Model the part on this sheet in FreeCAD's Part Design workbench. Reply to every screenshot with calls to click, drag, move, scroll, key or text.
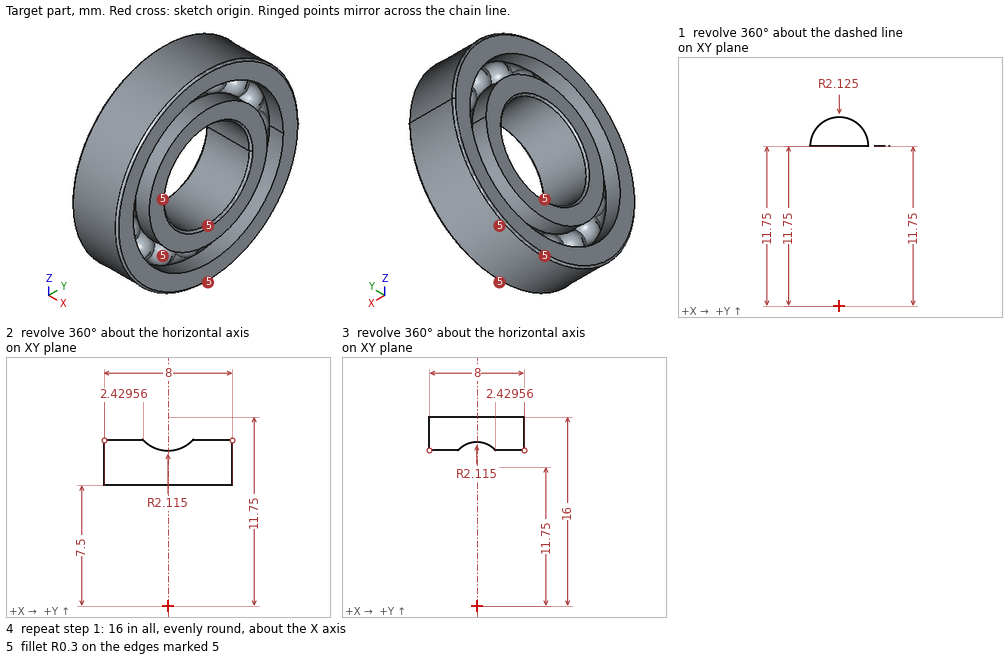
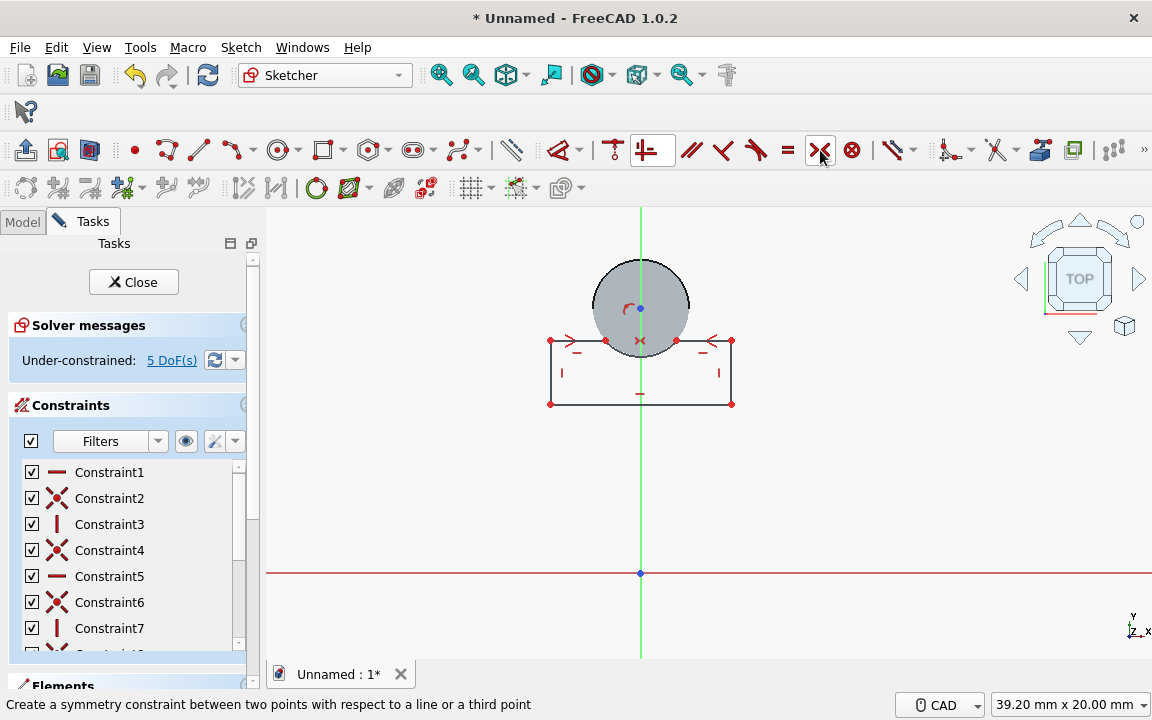
click(558, 150)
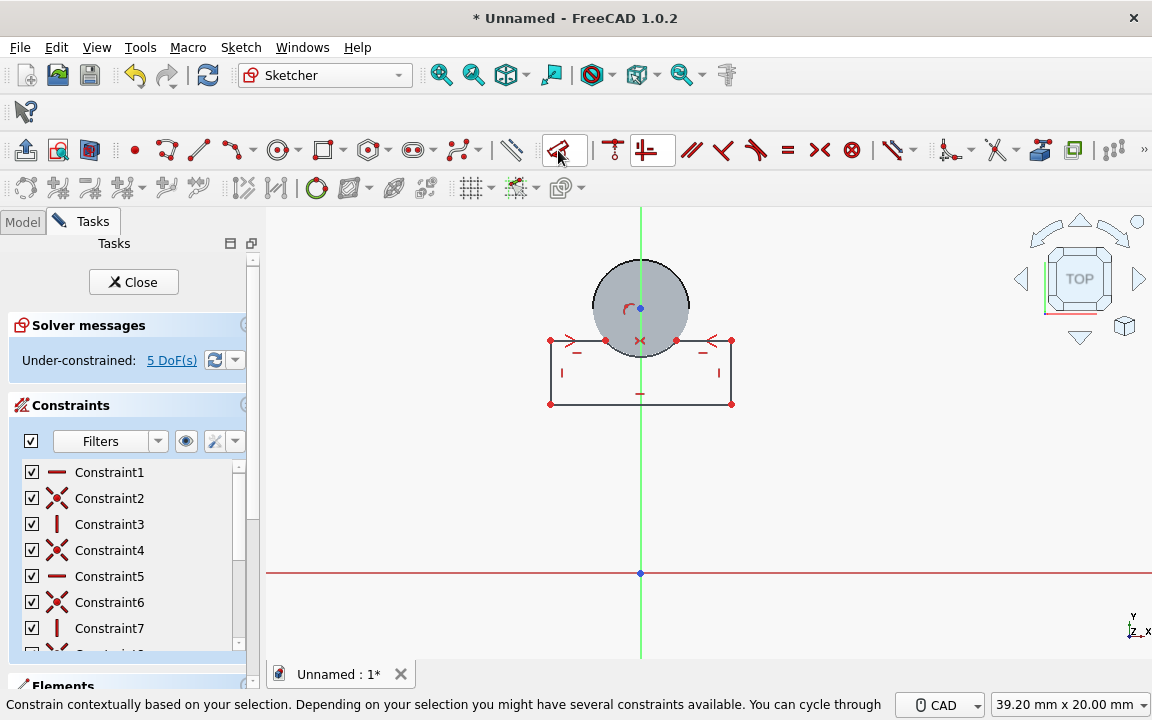
click(625, 354)
click(614, 384)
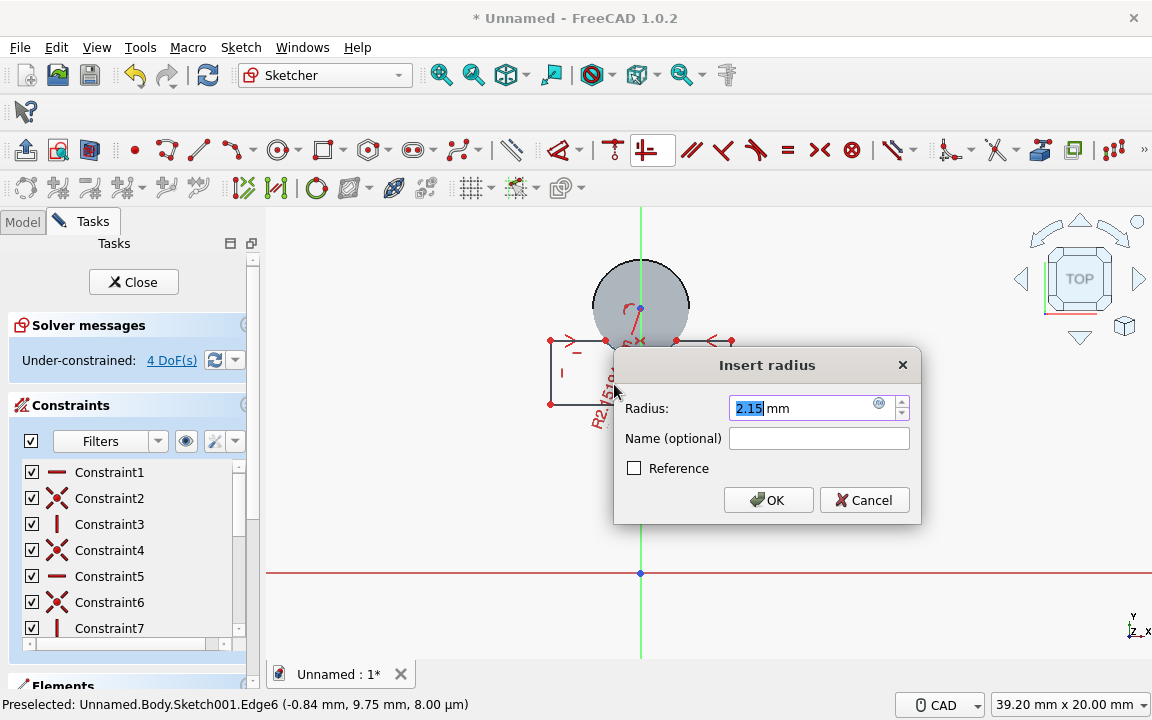
text(2.115)
key(Return)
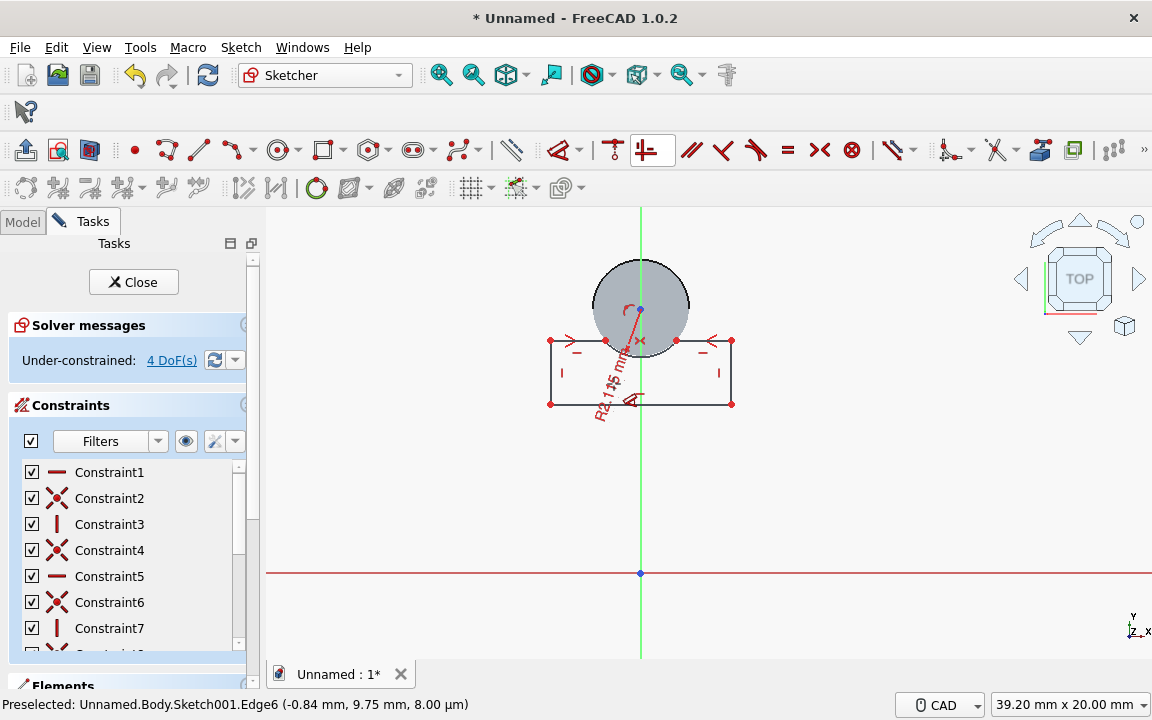
click(605, 405)
click(704, 371)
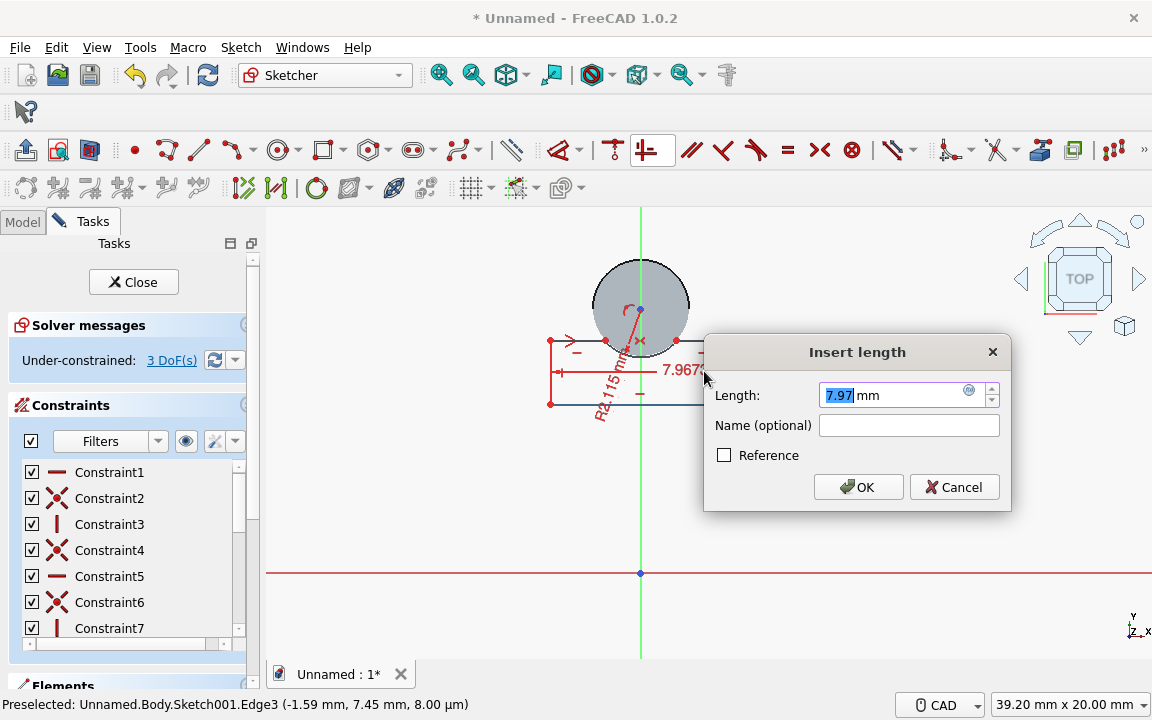
text(8)
key(Return)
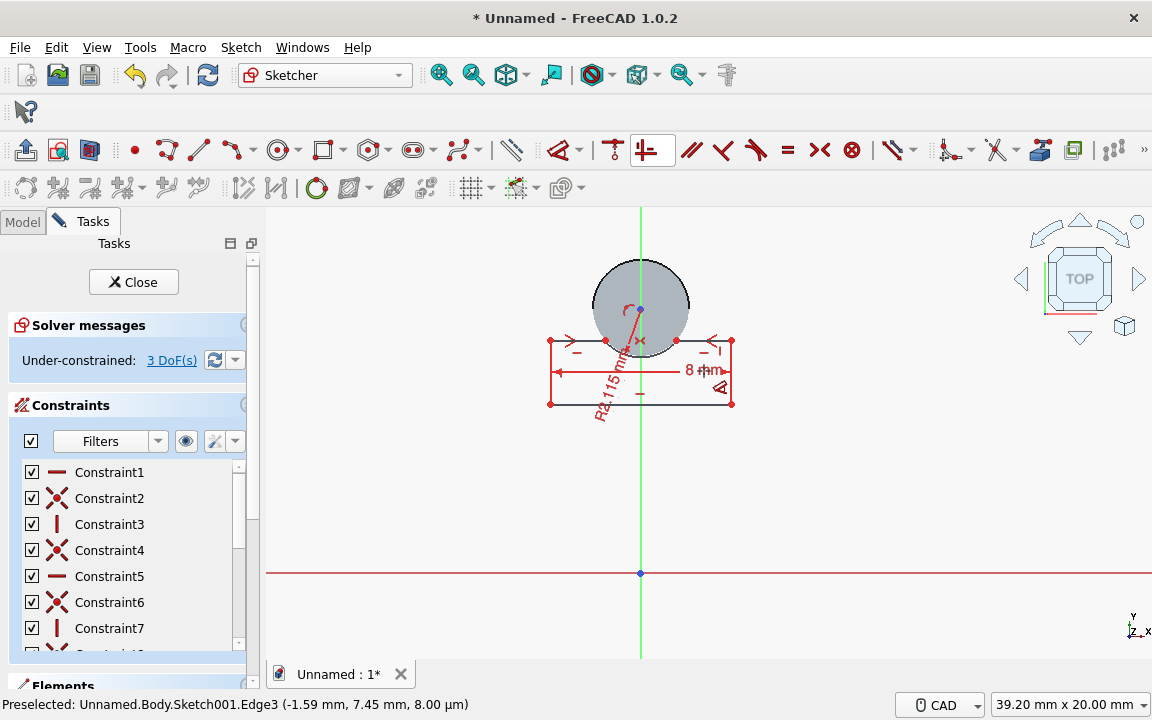
click(551, 405)
click(517, 489)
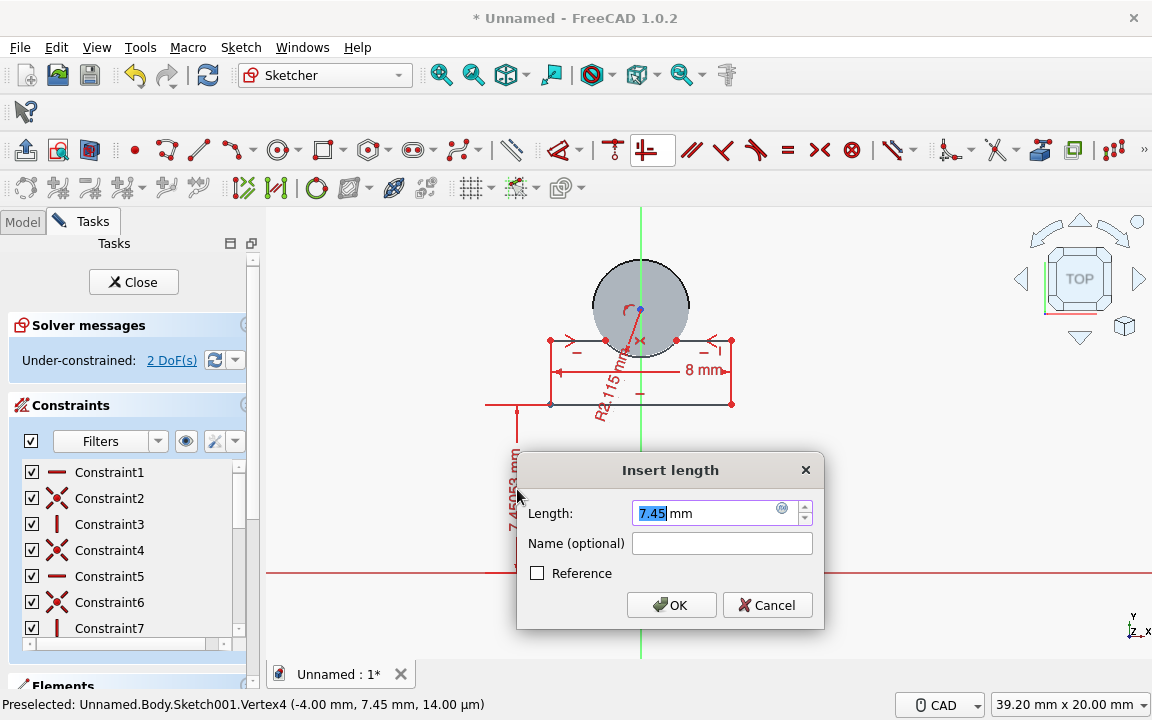
text(7.5)
key(Return)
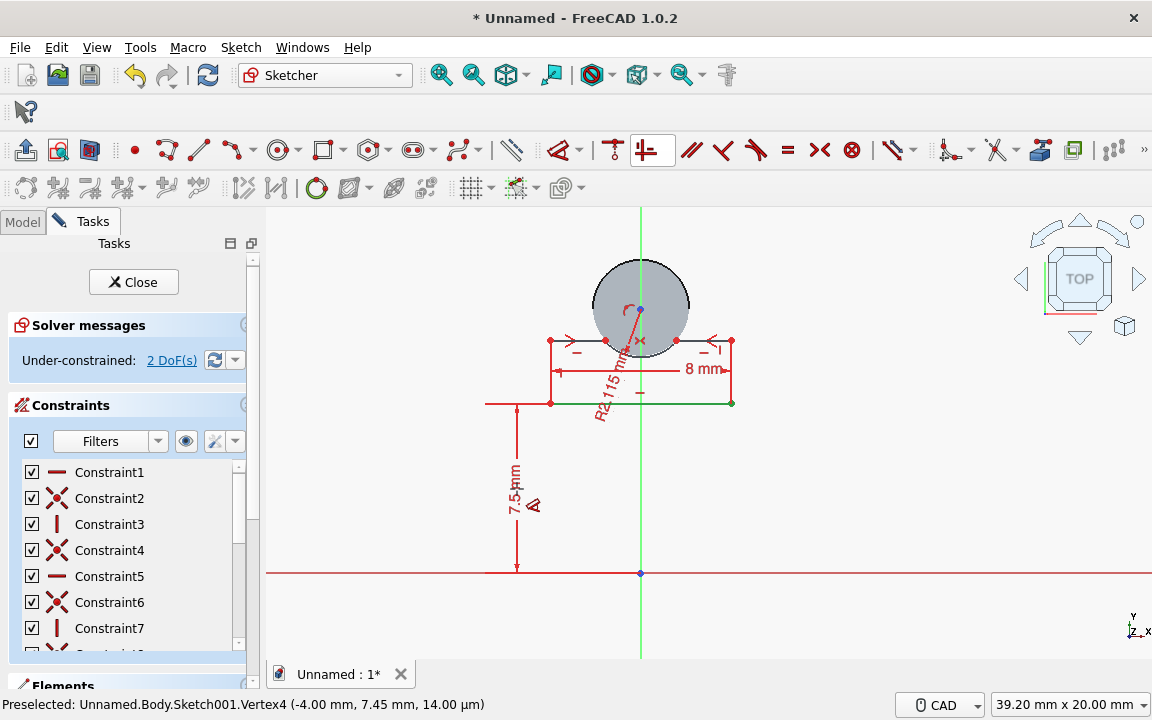
click(641, 310)
click(675, 441)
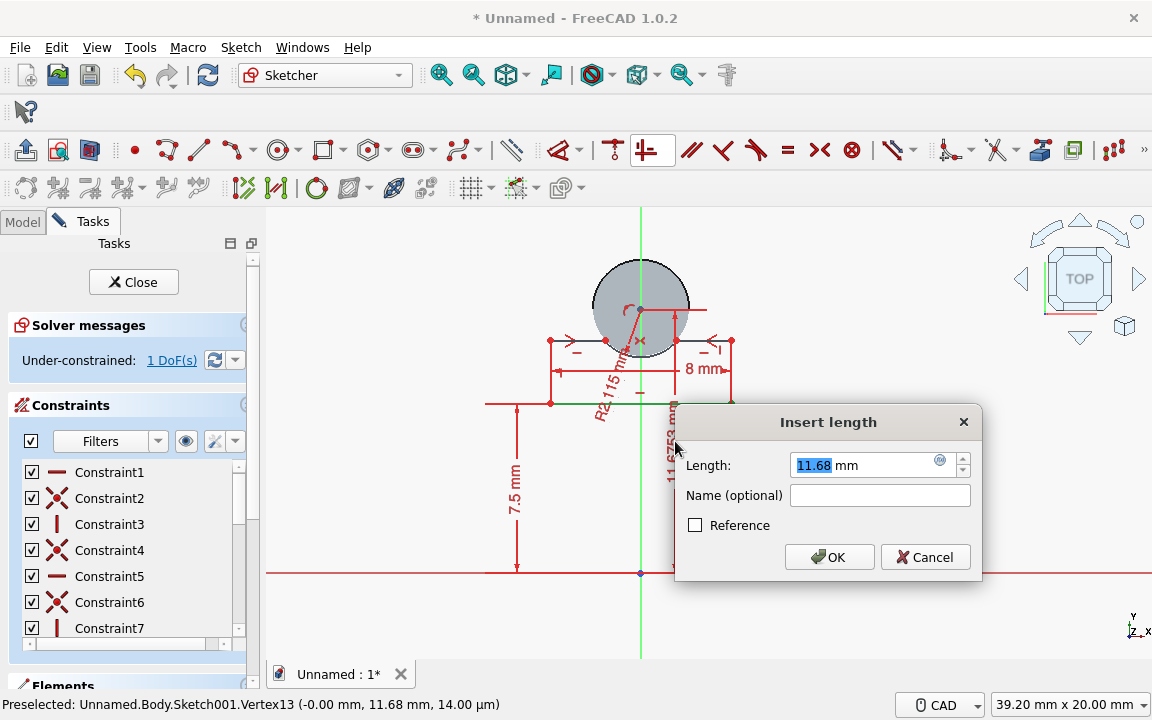
text(11.75)
key(Return)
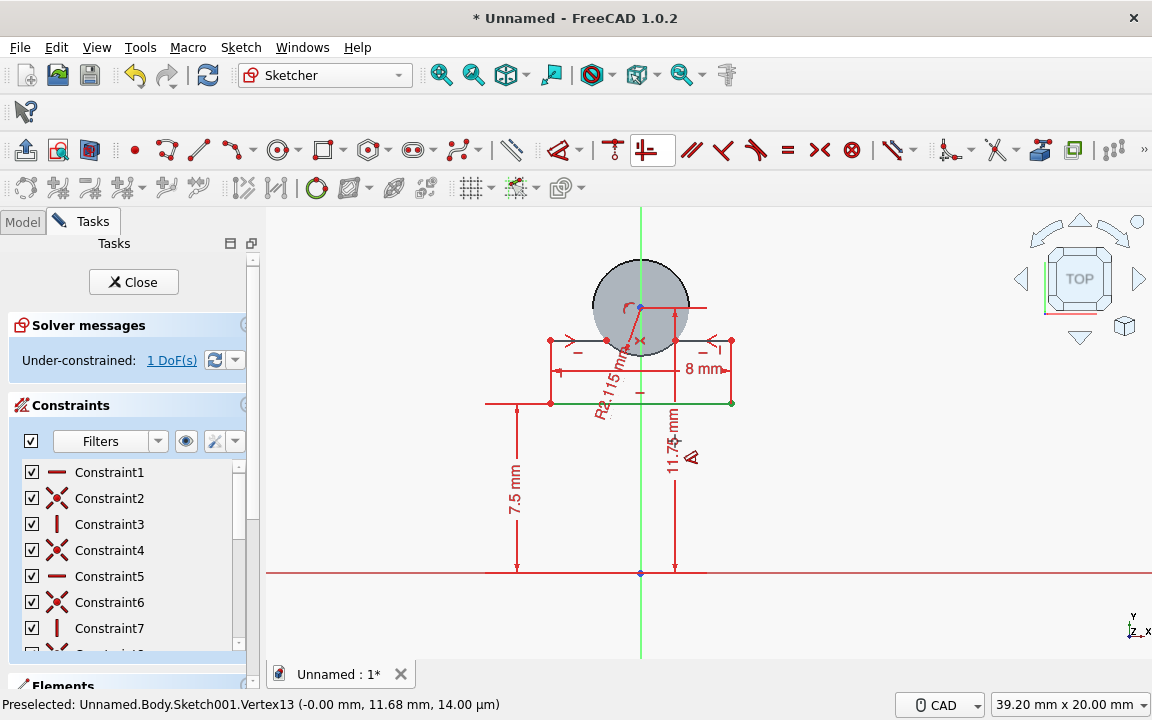
click(590, 341)
click(579, 307)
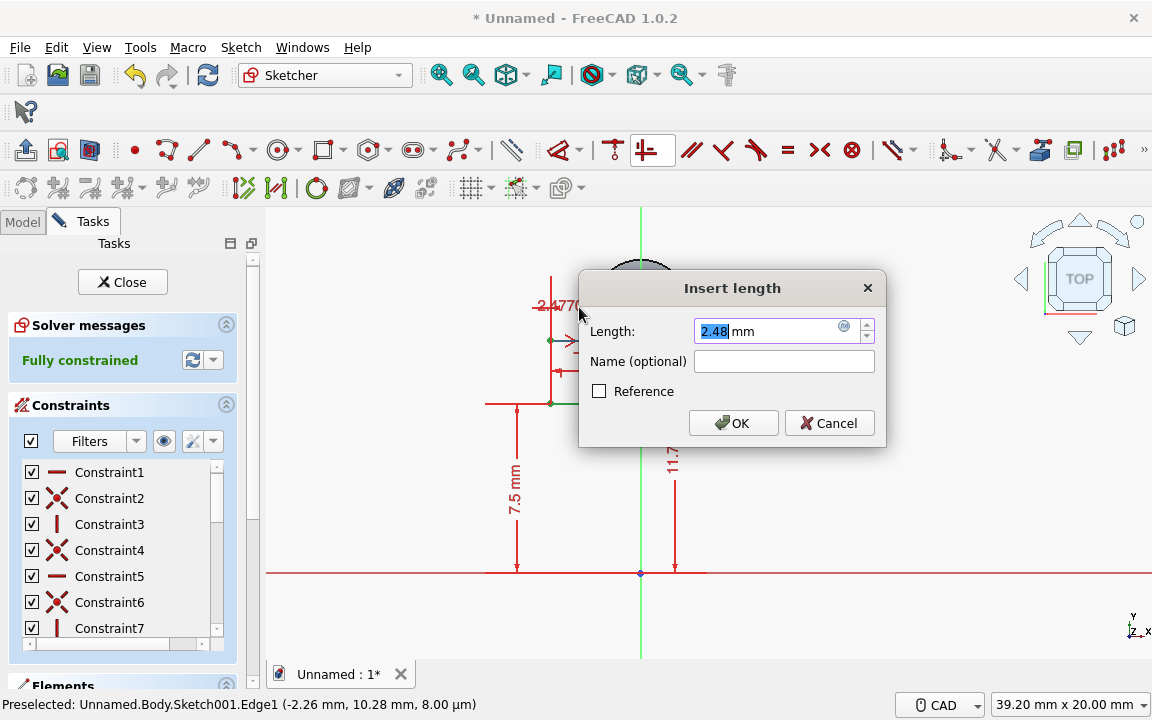
text(2.42956)
key(Return)
key(Escape)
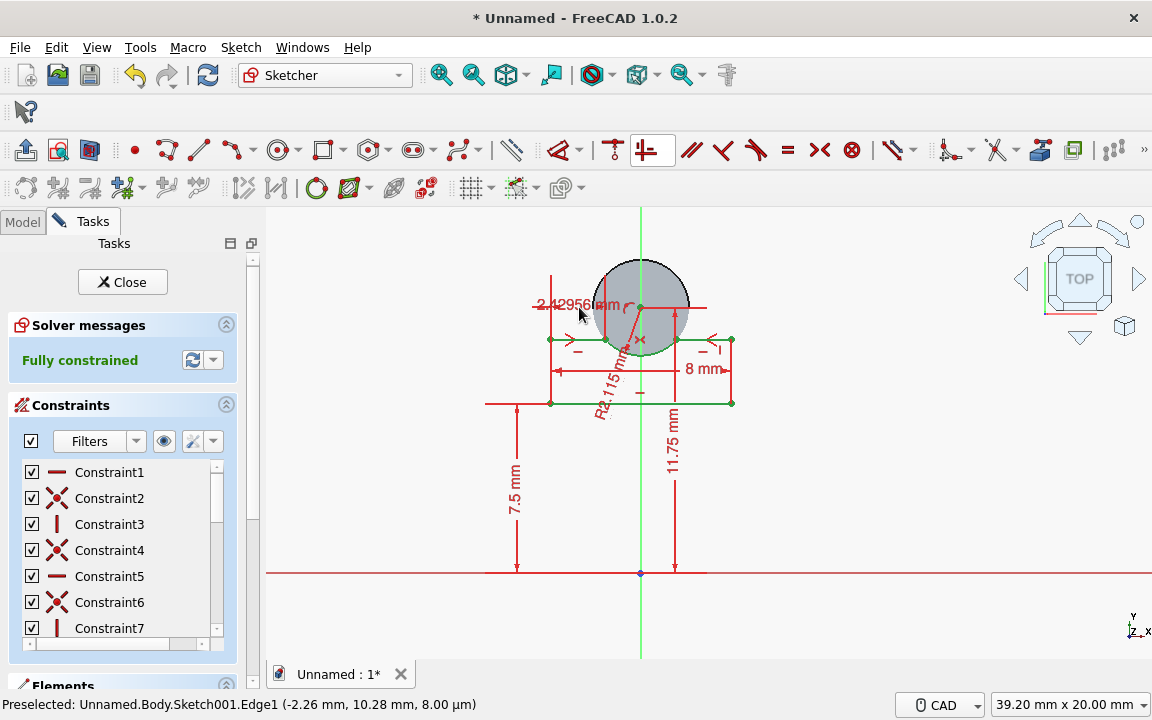
click(123, 282)